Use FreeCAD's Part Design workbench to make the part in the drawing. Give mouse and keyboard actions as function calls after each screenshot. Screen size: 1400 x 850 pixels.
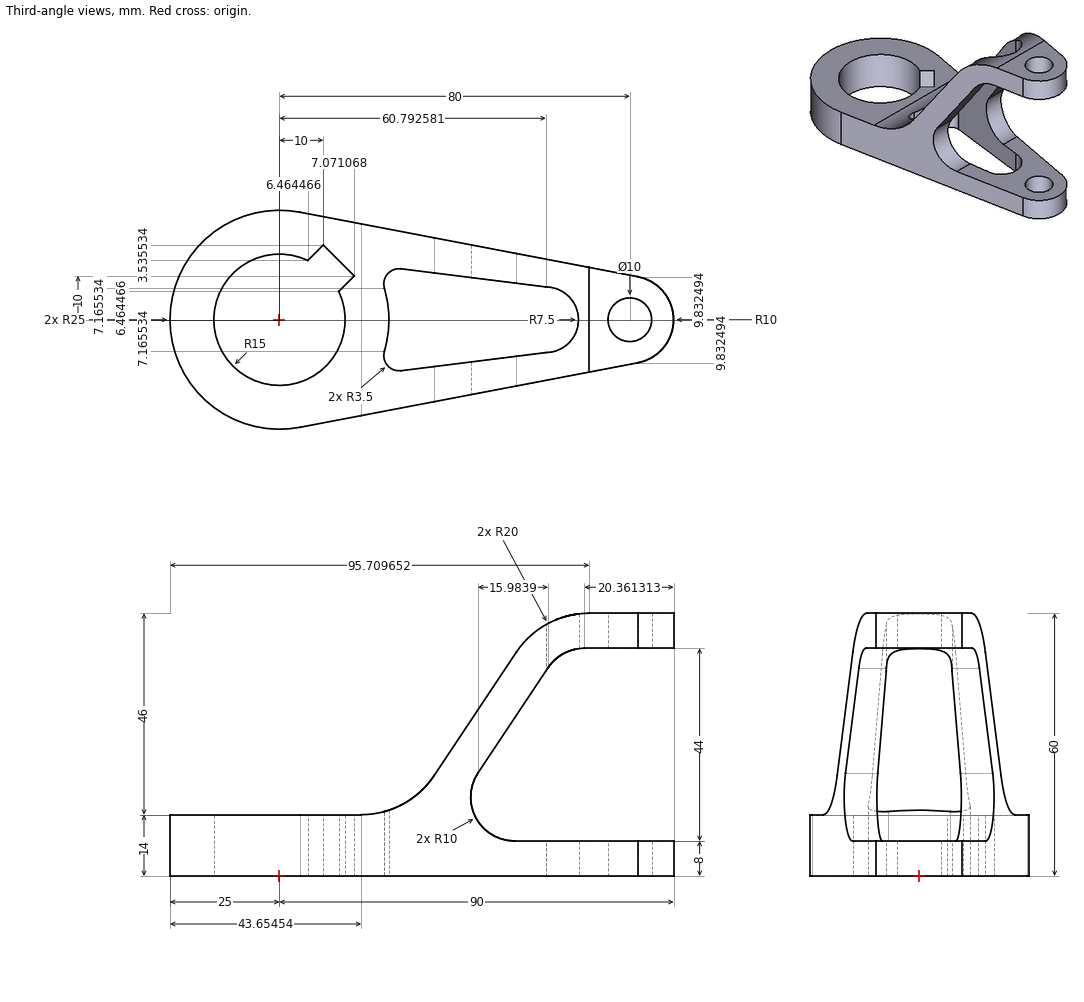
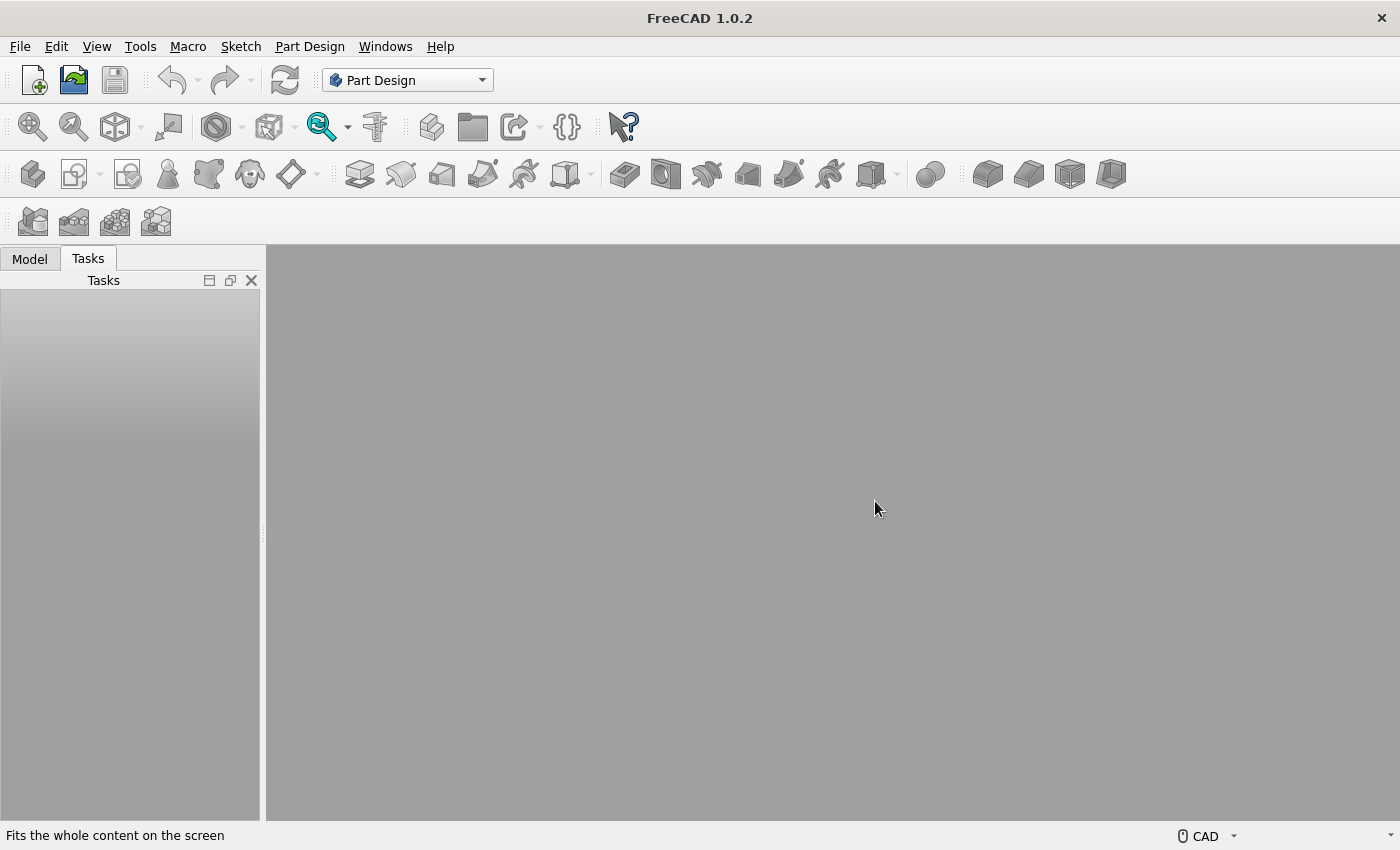
click(33, 80)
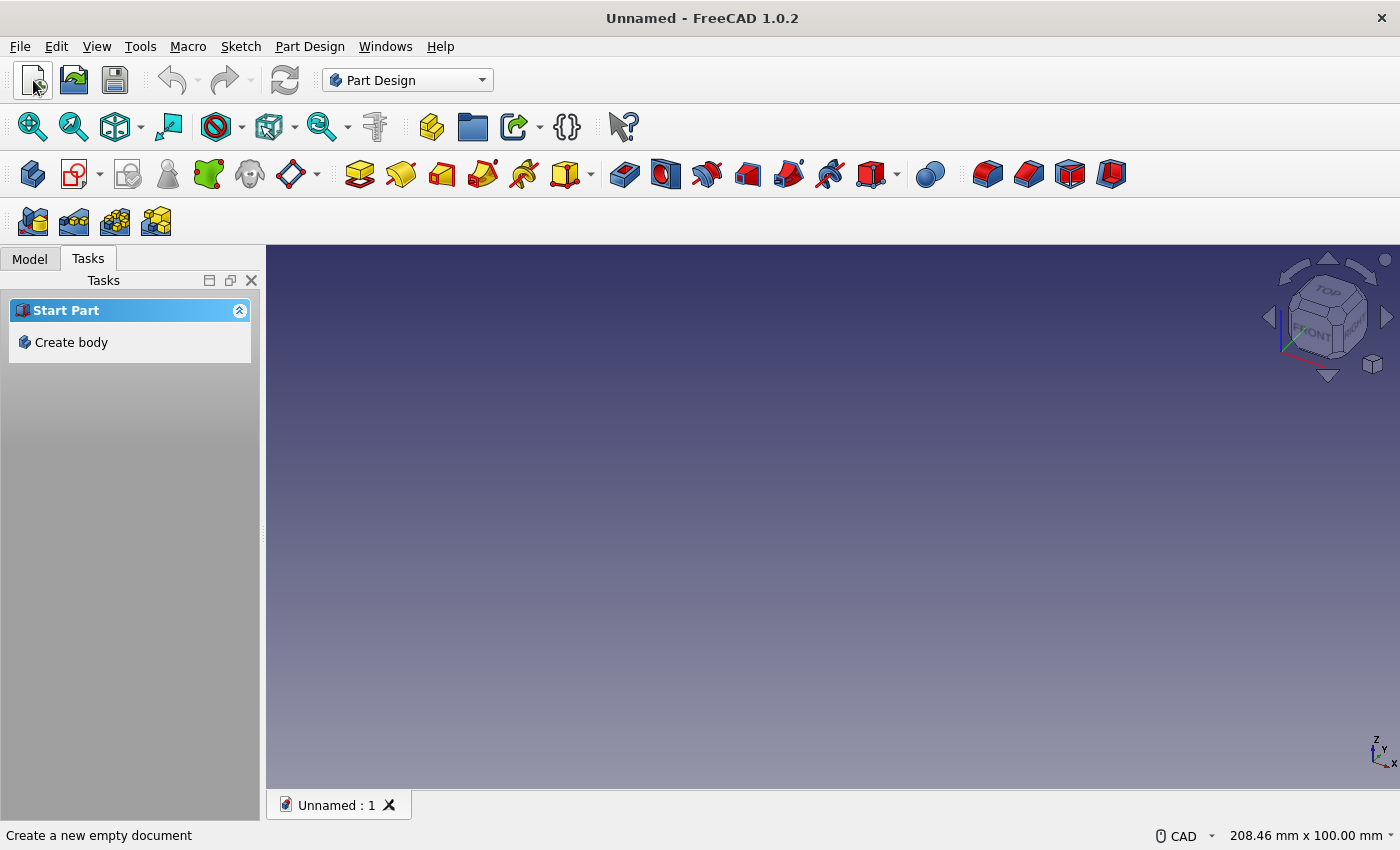
click(74, 174)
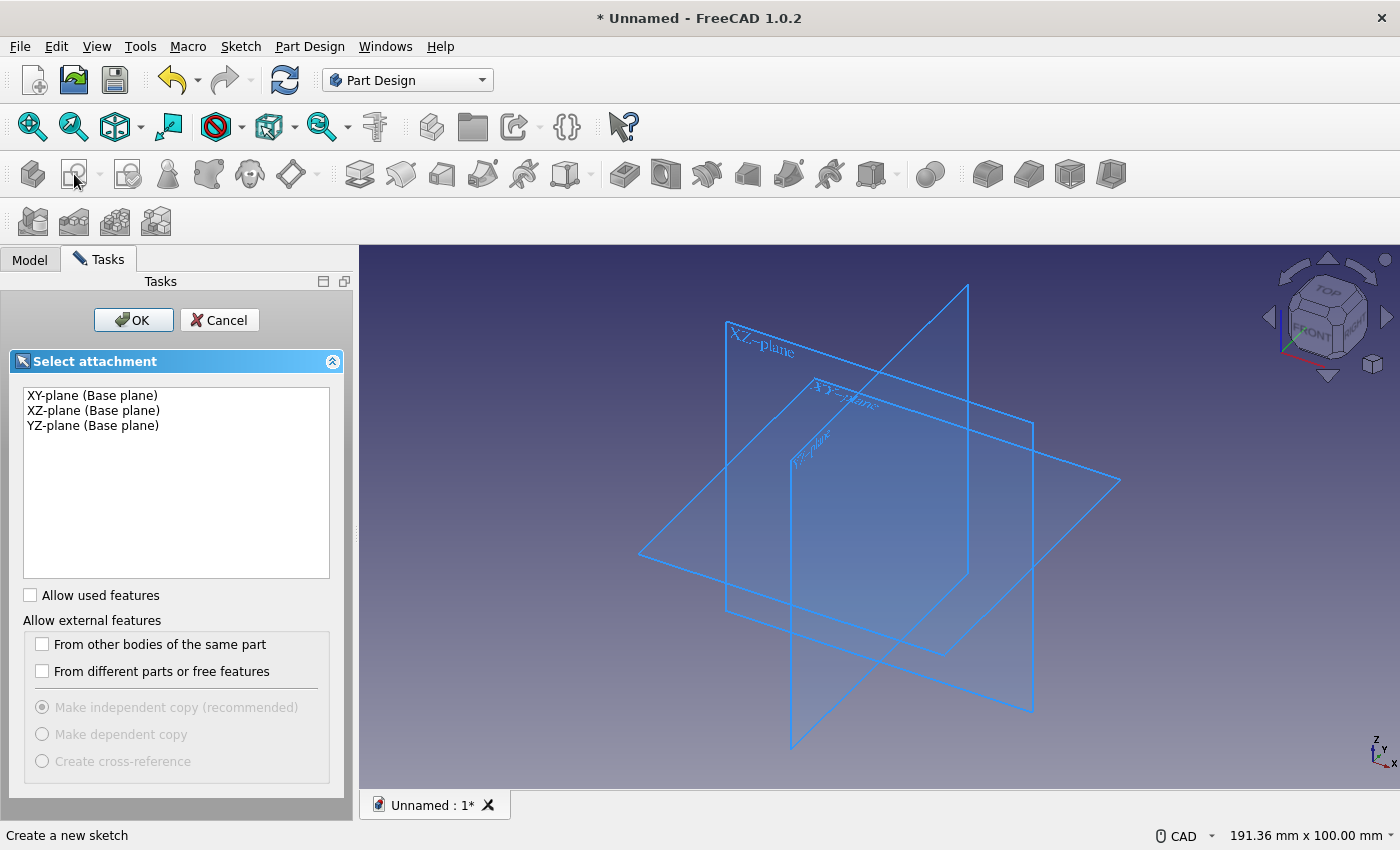
click(84, 396)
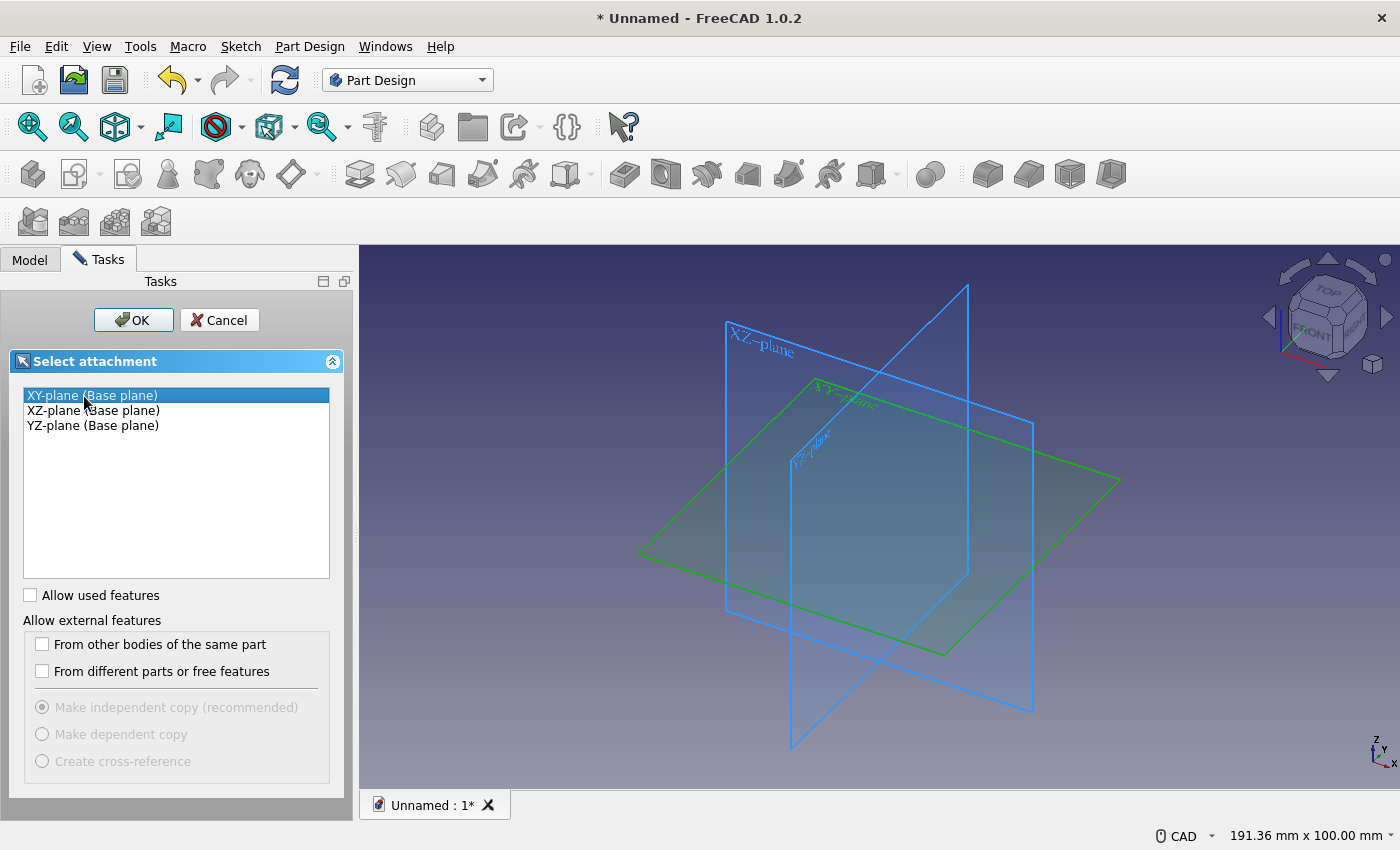
click(134, 320)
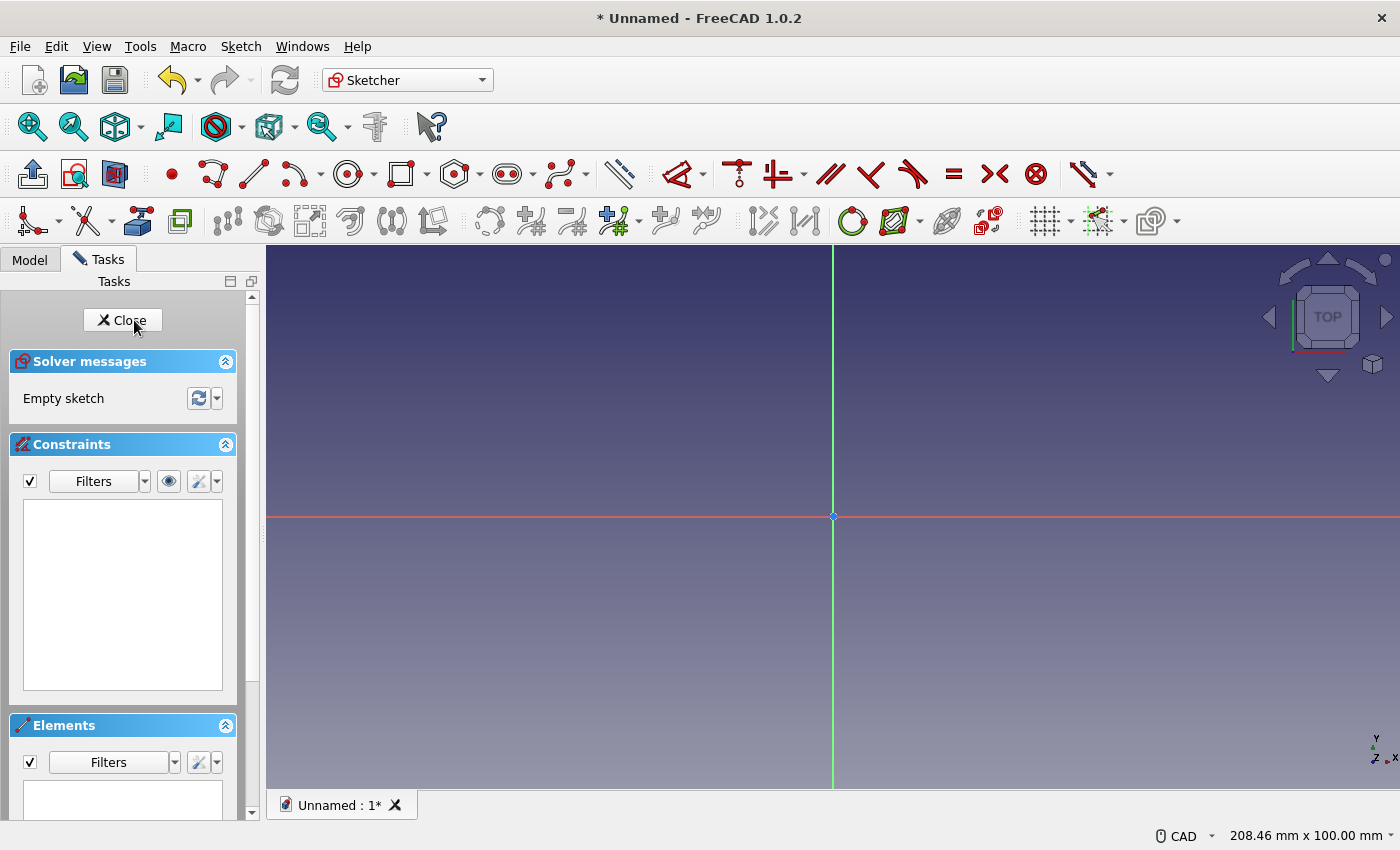
scroll(294, 517, down, 1)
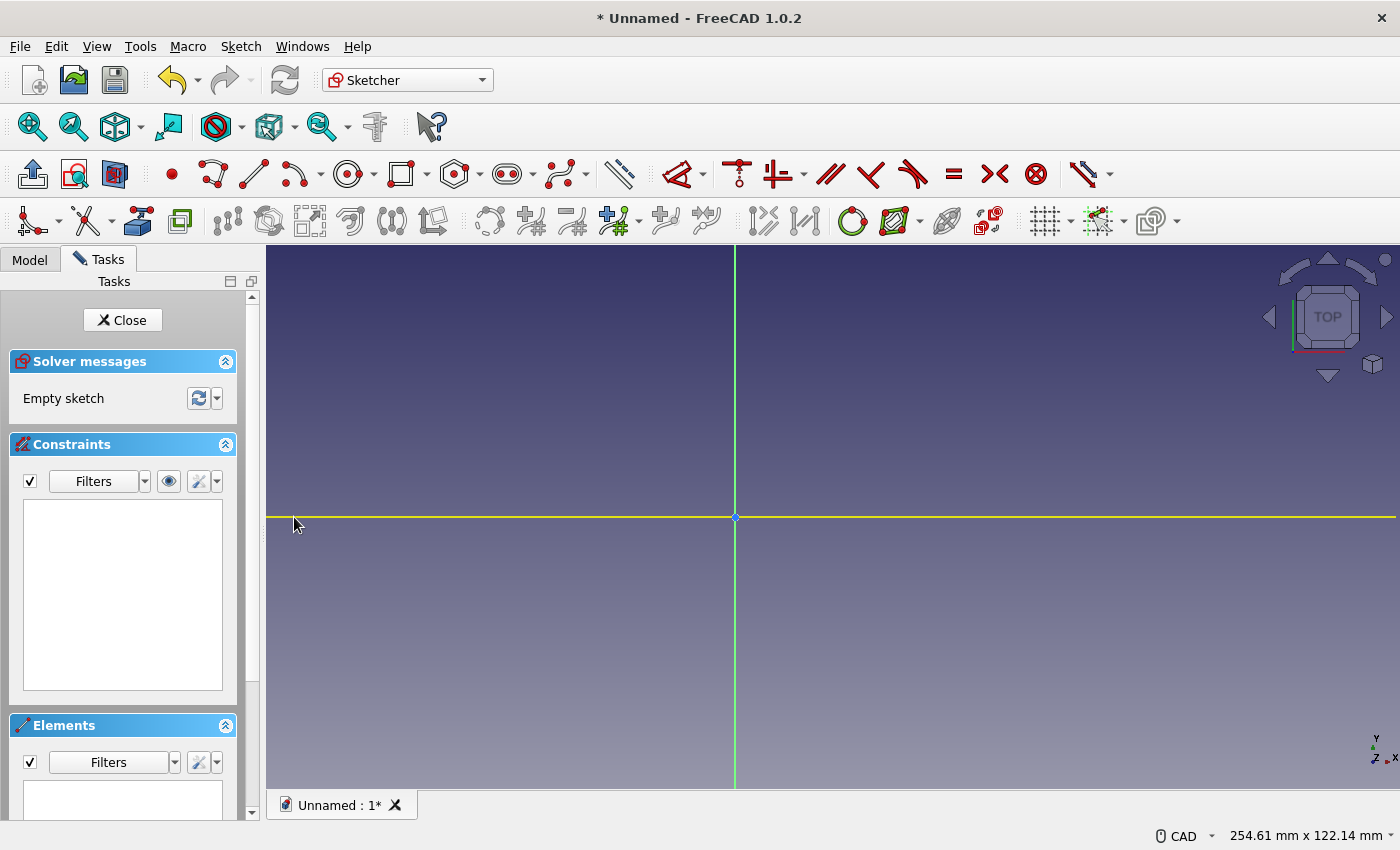
click(254, 174)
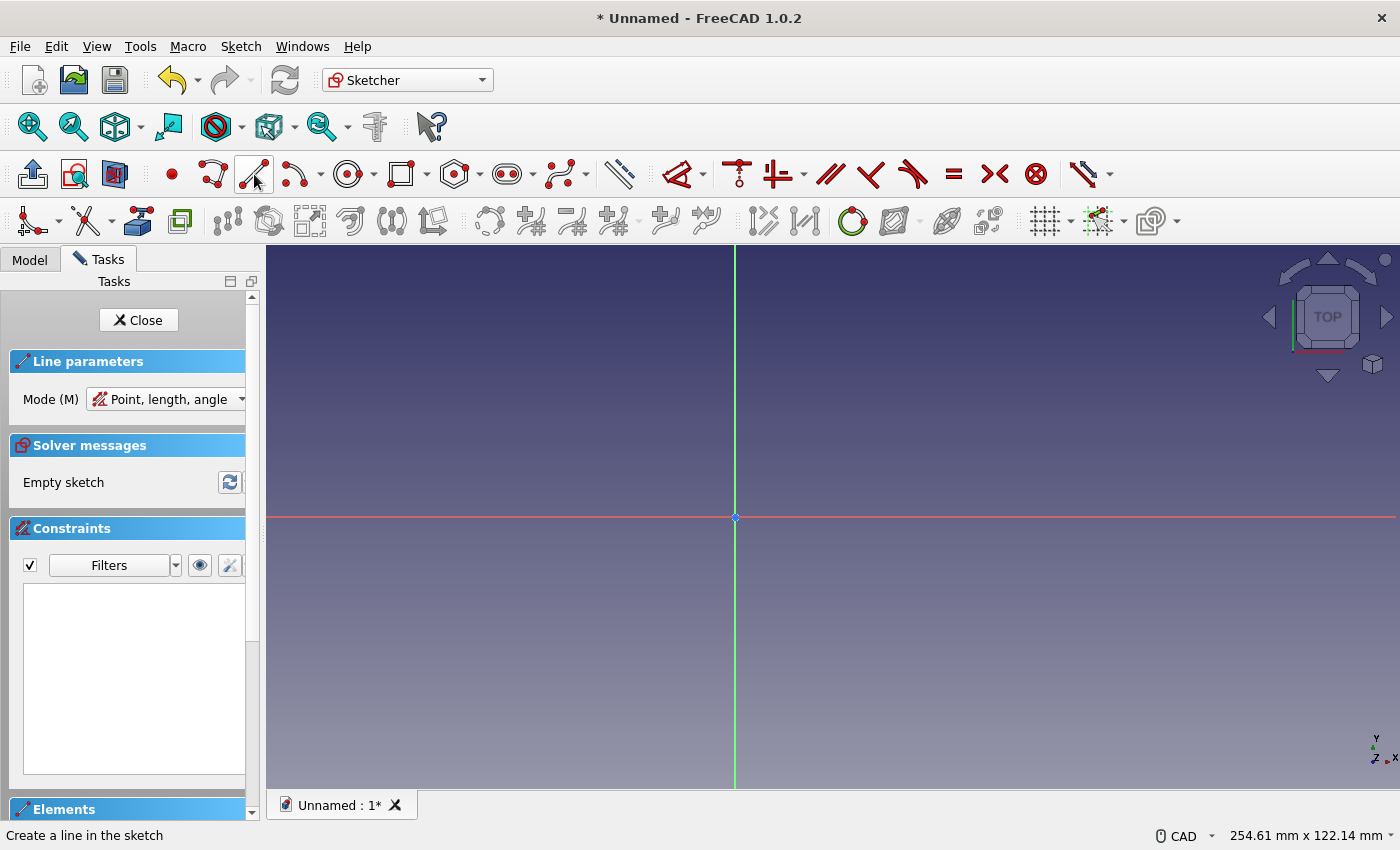
click(1100, 473)
click(756, 408)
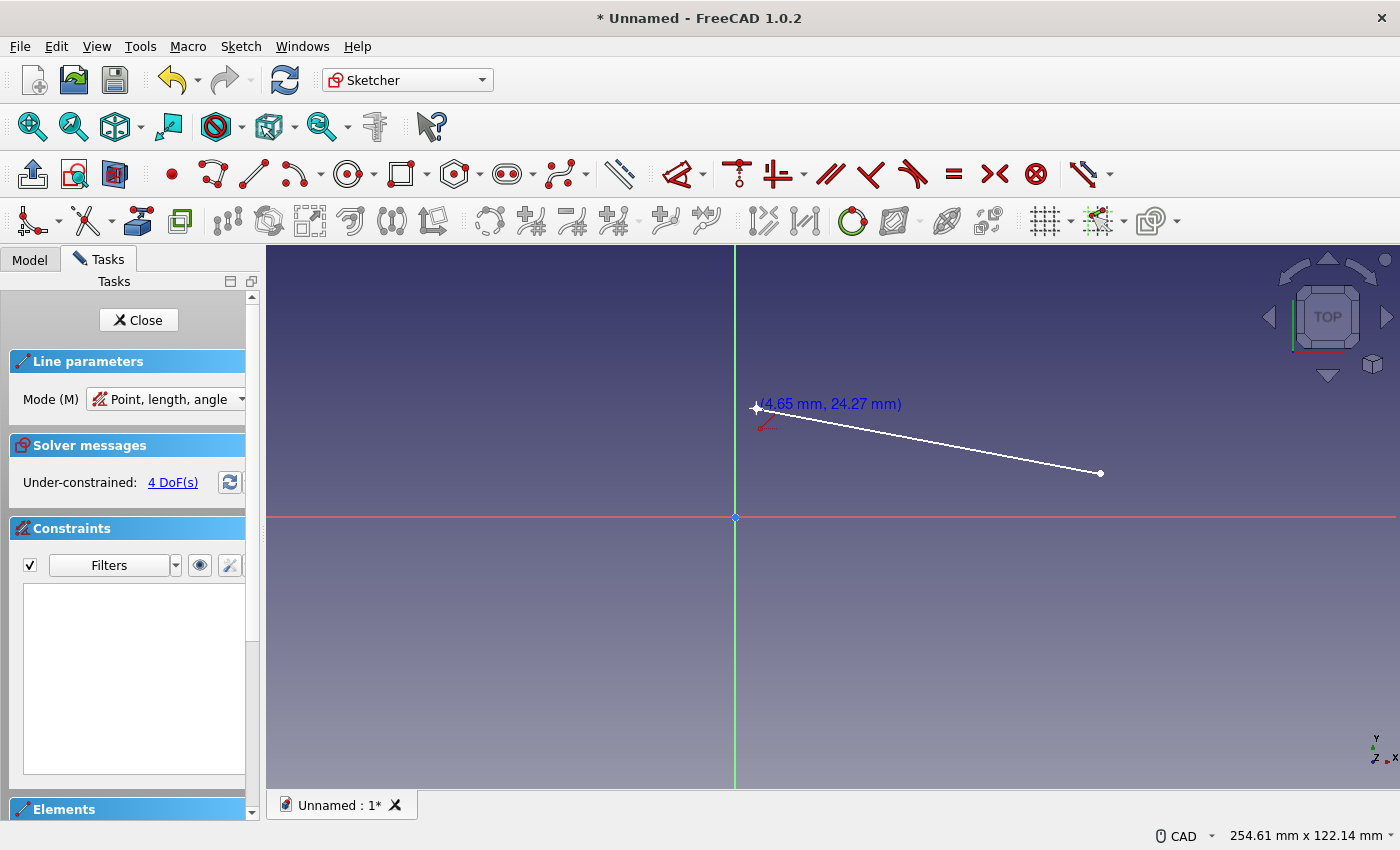
click(756, 626)
click(1100, 561)